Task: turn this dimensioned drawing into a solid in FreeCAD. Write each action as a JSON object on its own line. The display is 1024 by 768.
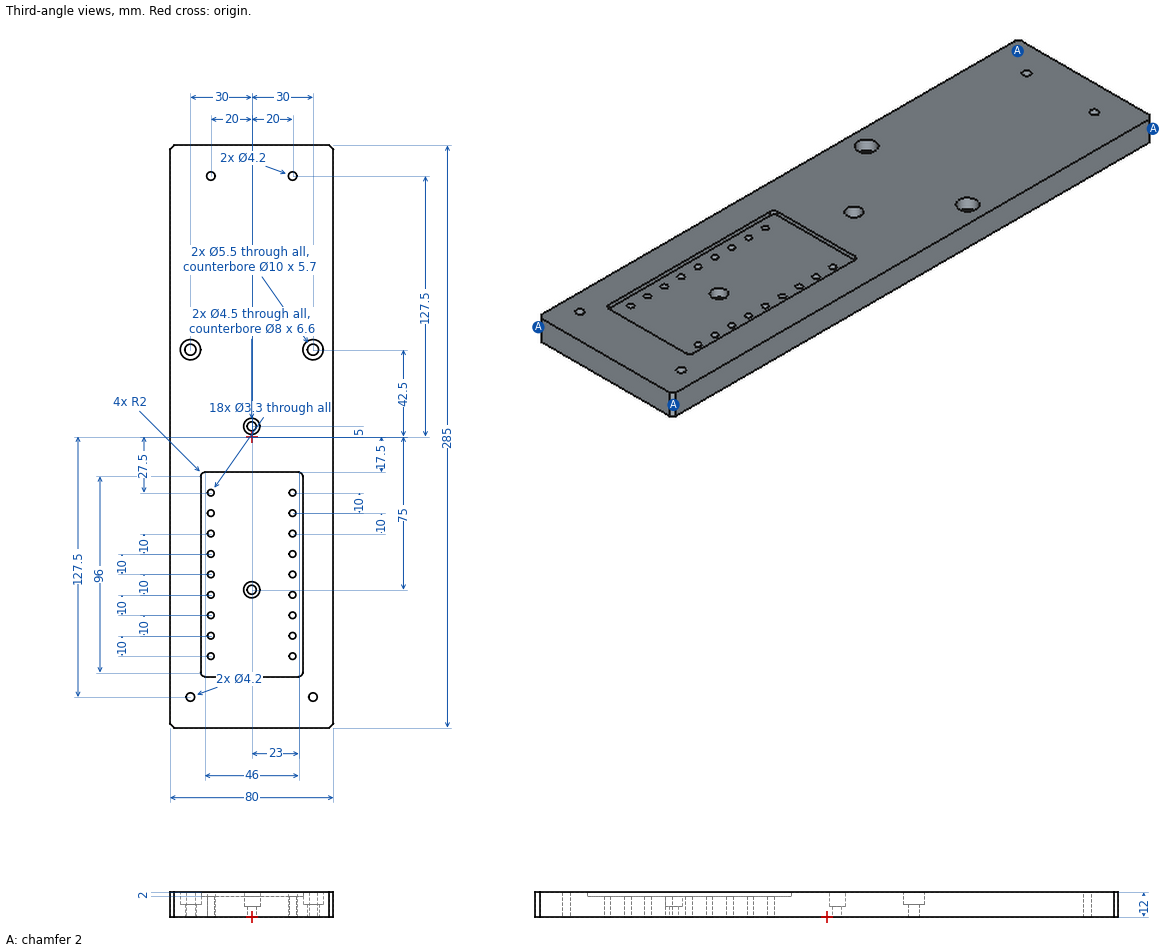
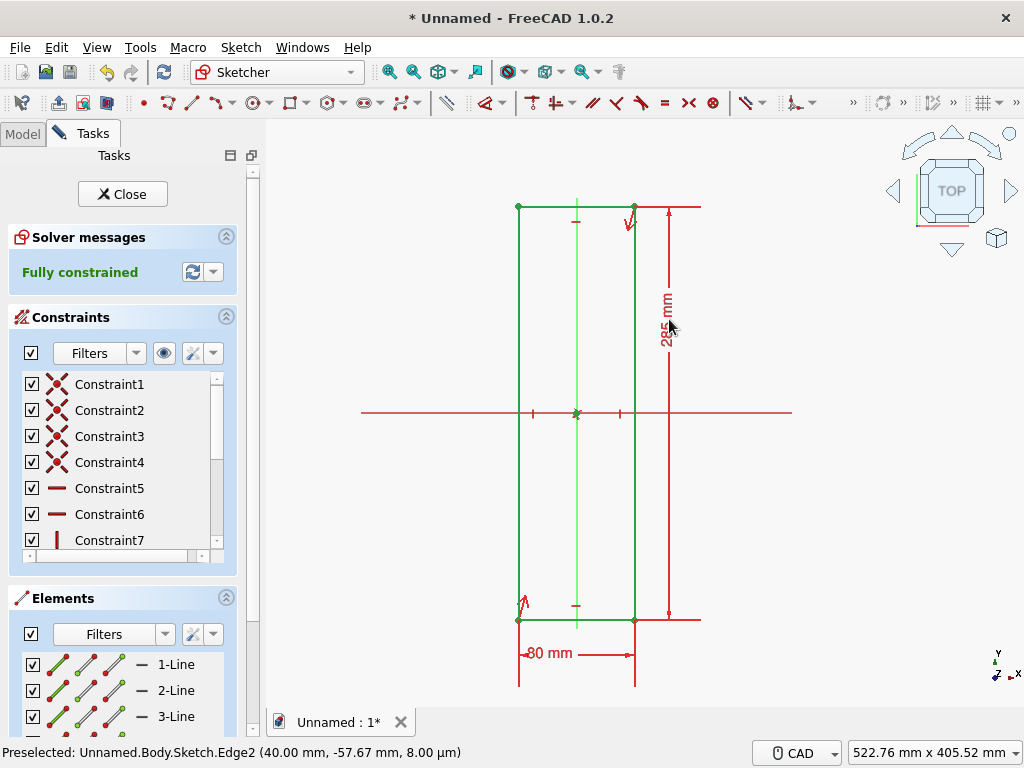
{"action": "left_click", "coordinate": [123, 194]}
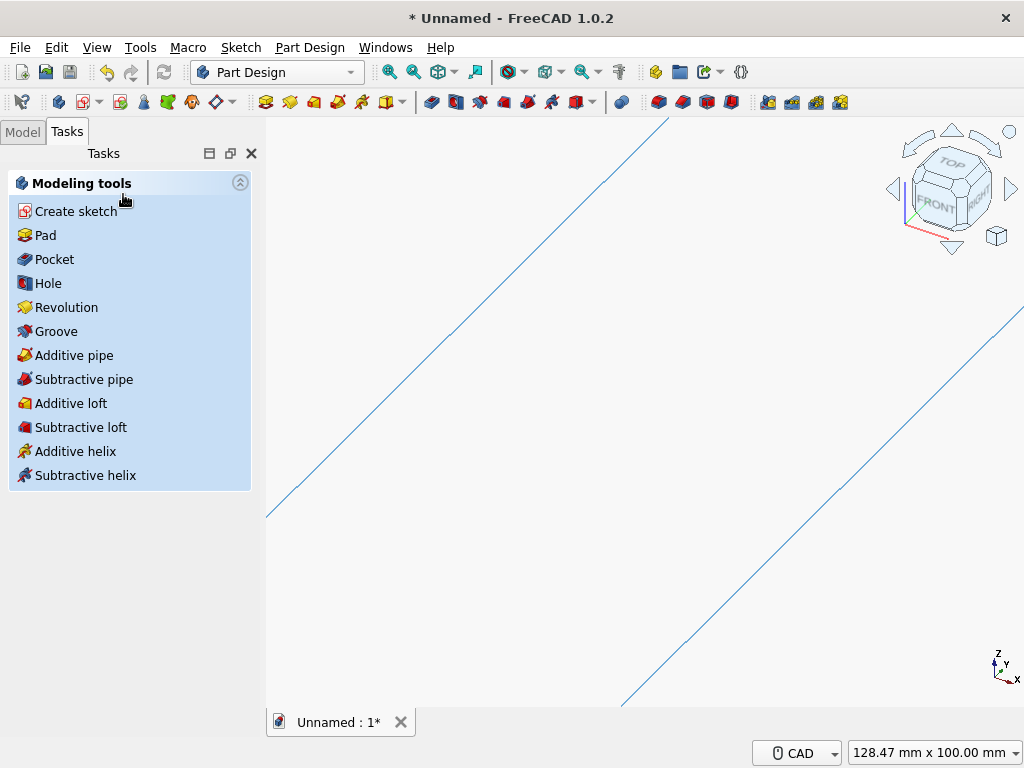
{"action": "left_click", "coordinate": [266, 102]}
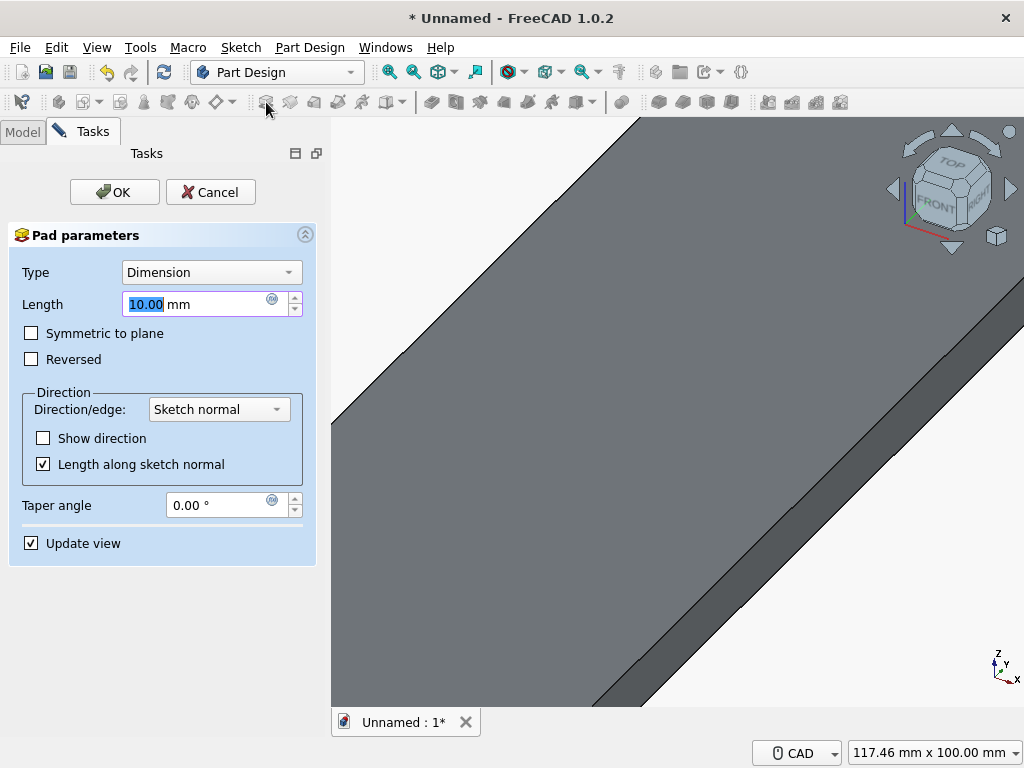
{"action": "type", "text": "12"}
{"action": "key", "text": "Tab"}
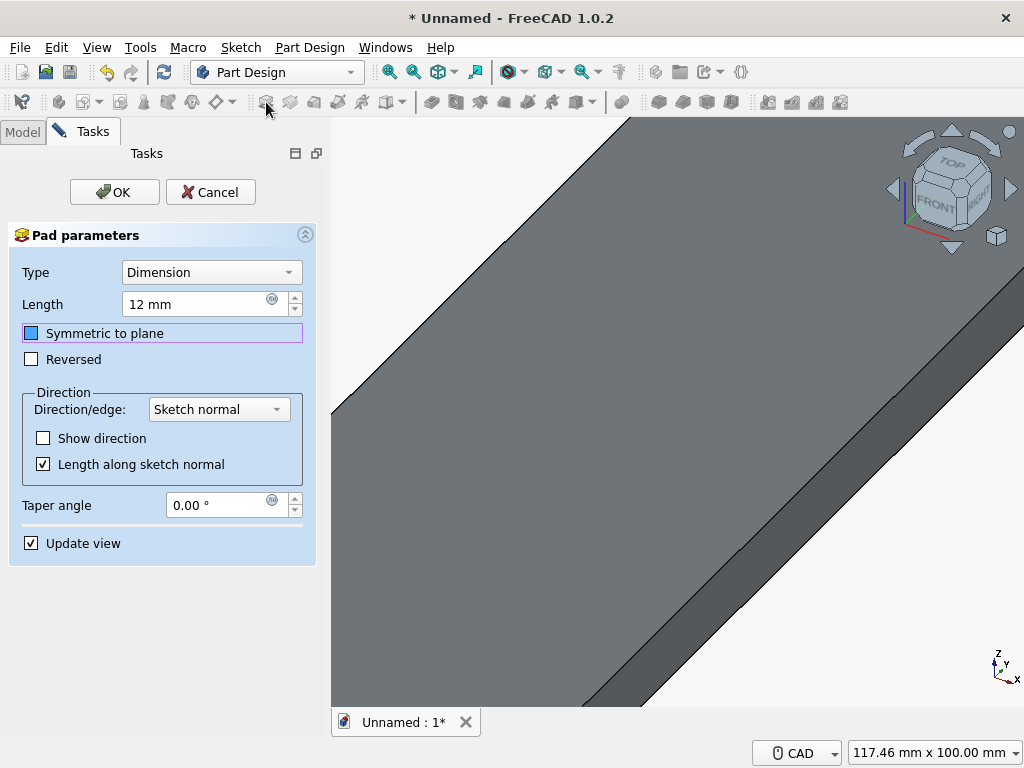
{"action": "left_click", "coordinate": [115, 192]}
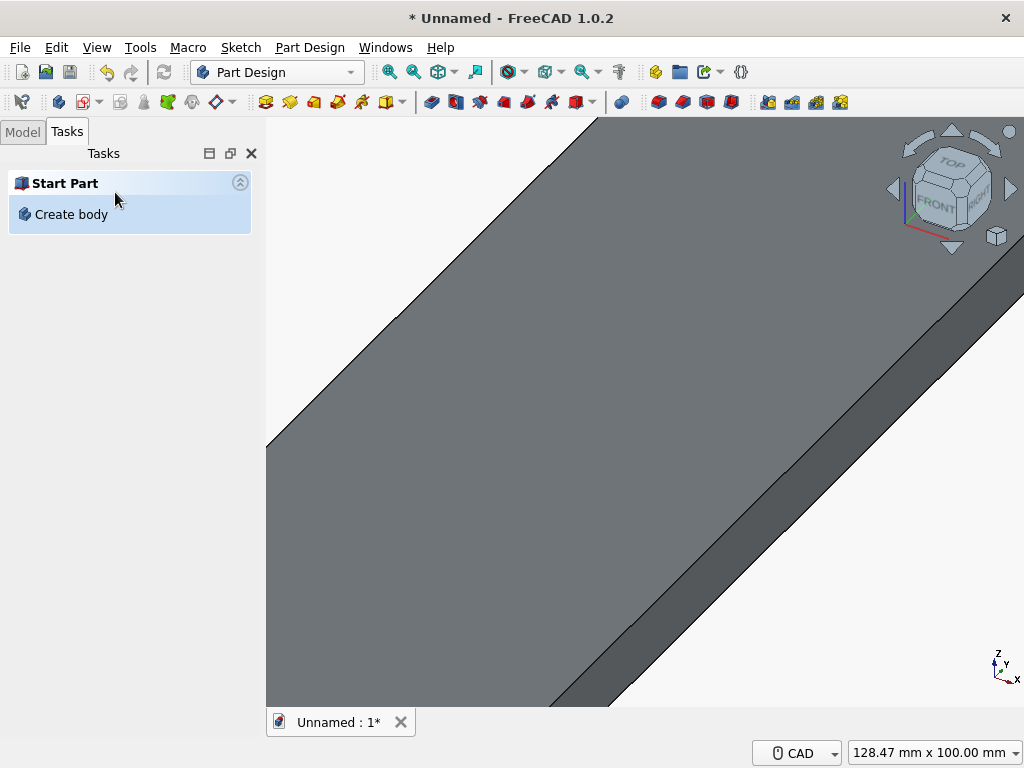
{"action": "left_click", "coordinate": [390, 72]}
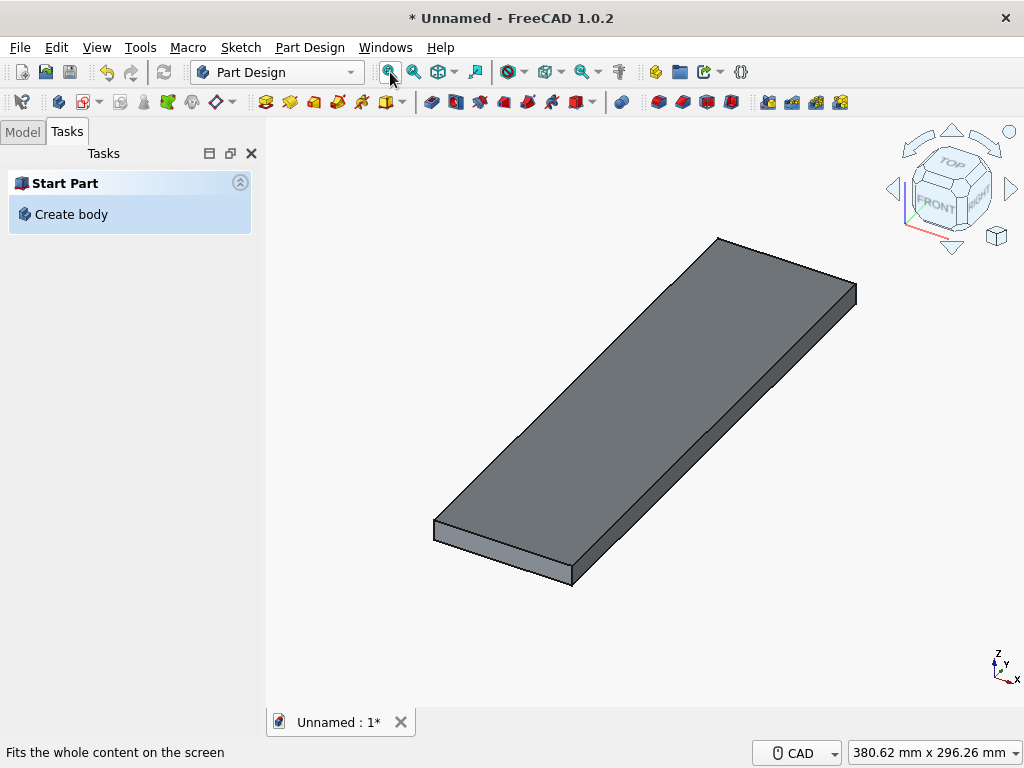
{"action": "left_click", "coordinate": [726, 321]}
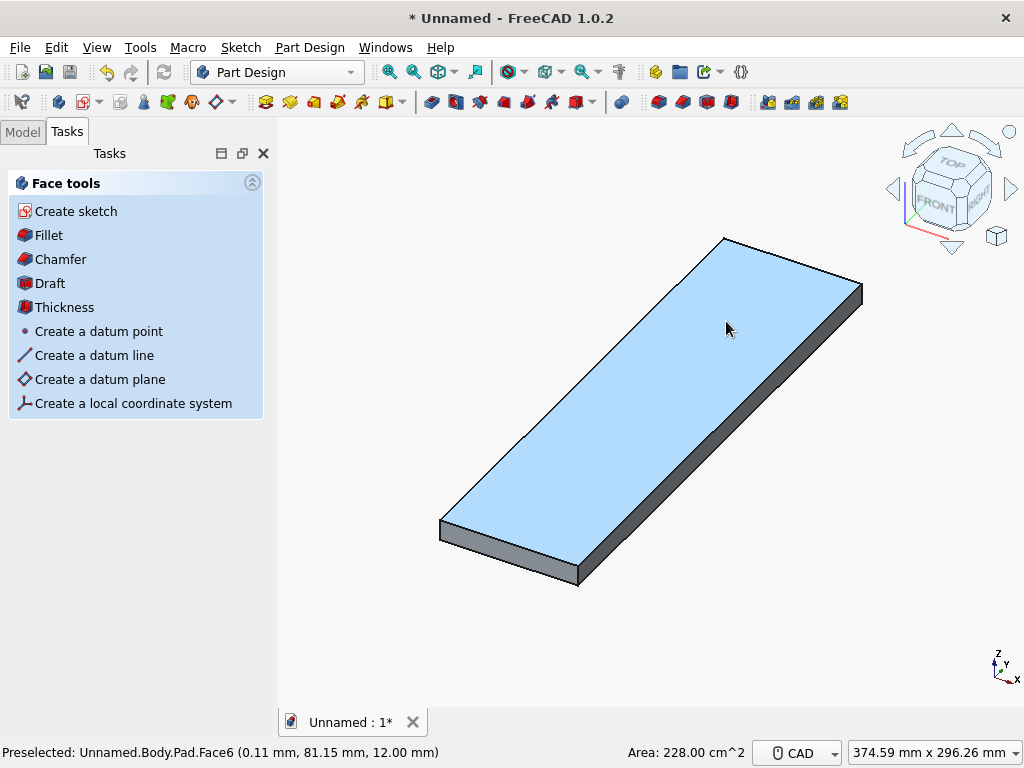
{"action": "left_click", "coordinate": [84, 102]}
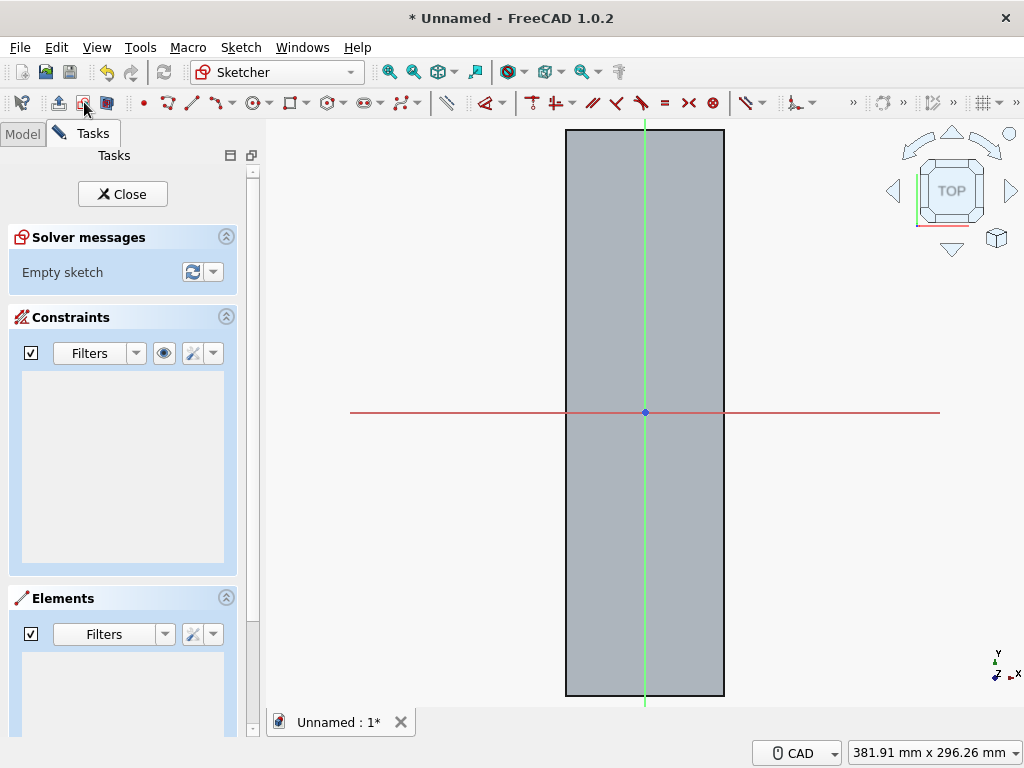
{"action": "scroll", "coordinate": [675, 349], "scroll_direction": "up", "scroll_amount": 6}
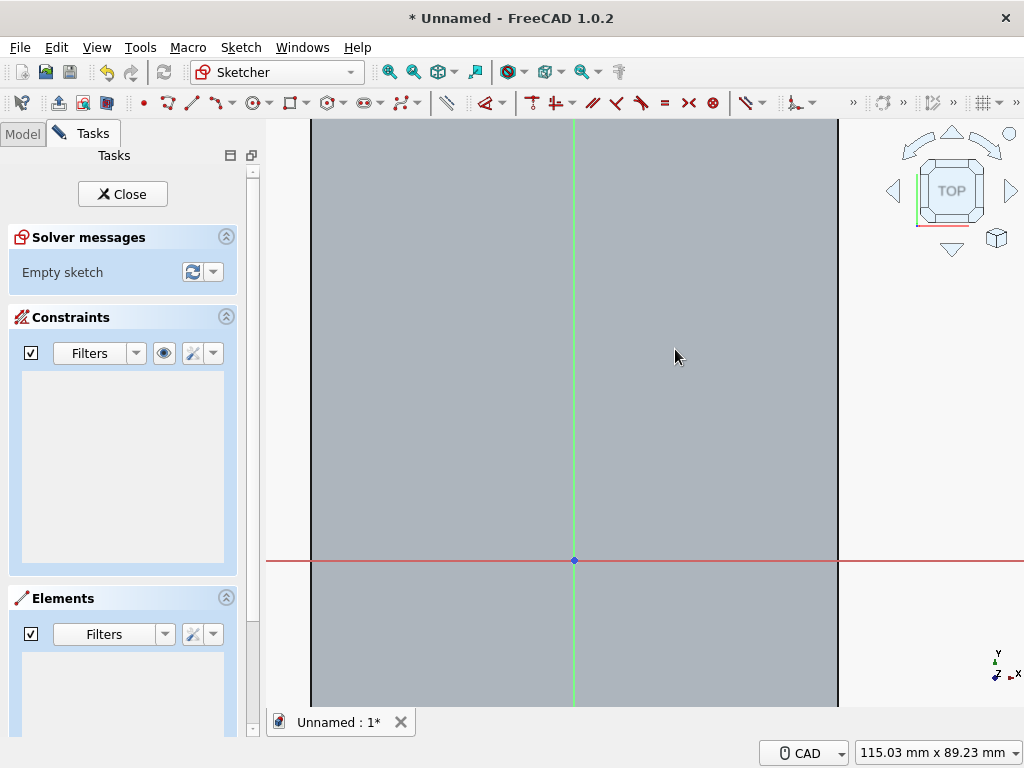
{"action": "key", "text": "g c"}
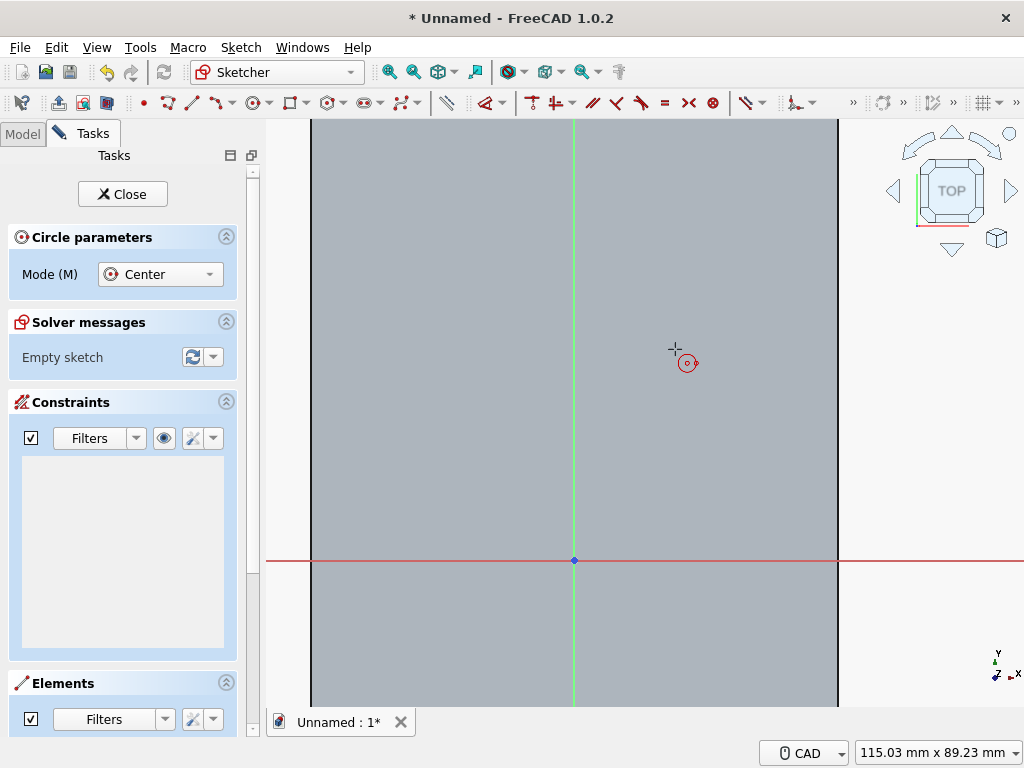
{"action": "scroll", "coordinate": [772, 281], "scroll_direction": "up", "scroll_amount": 2}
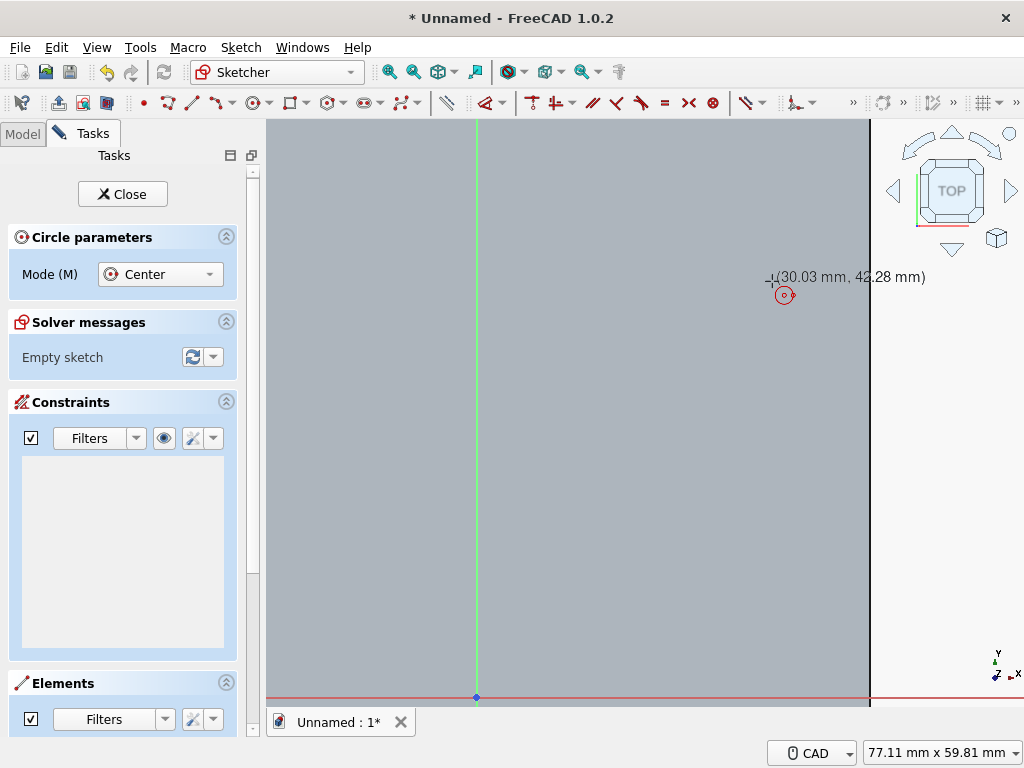
{"action": "left_click", "coordinate": [771, 280]}
{"action": "left_click", "coordinate": [791, 261]}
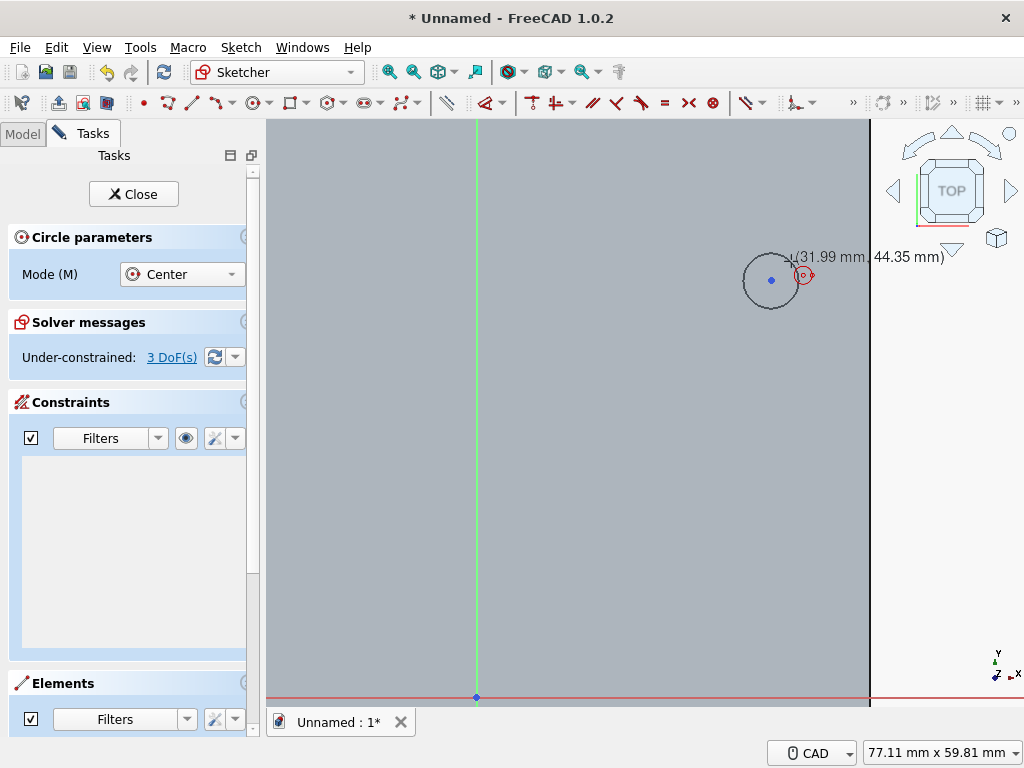
{"action": "scroll", "coordinate": [780, 286], "scroll_direction": "down", "scroll_amount": 2}